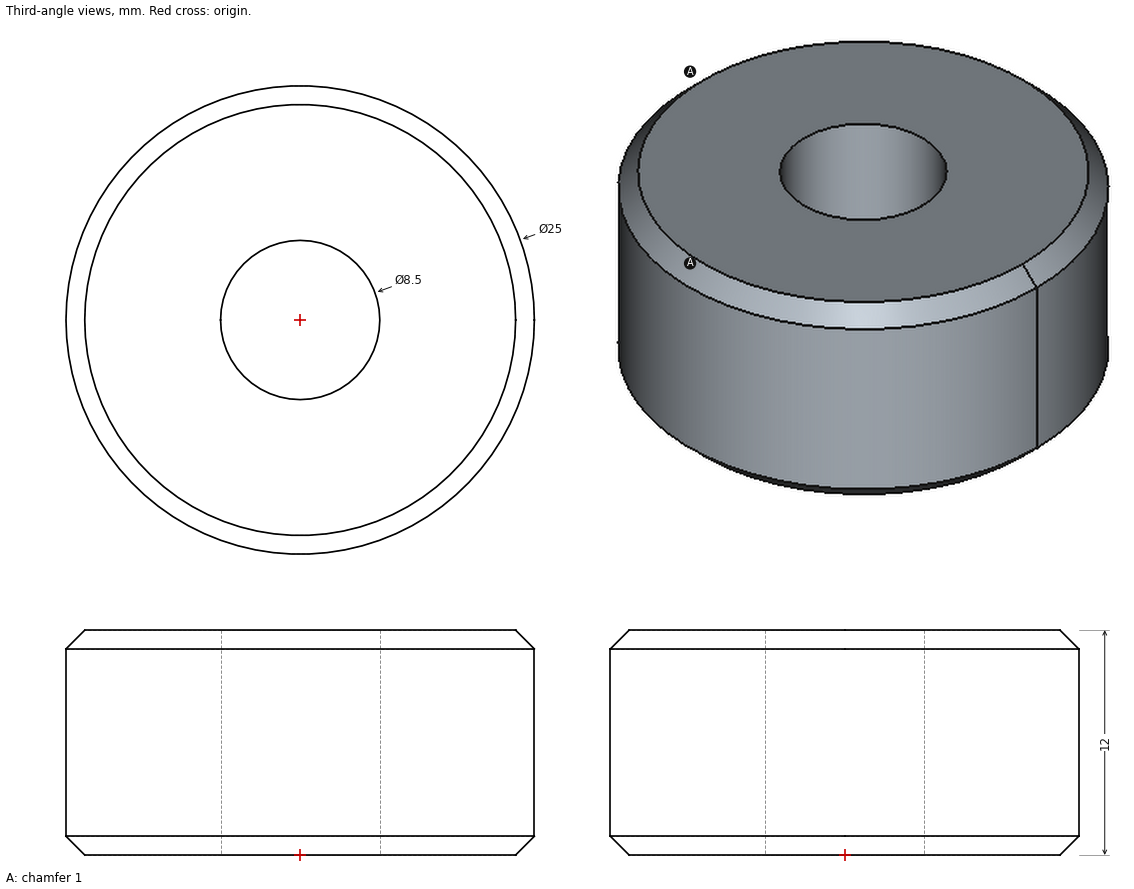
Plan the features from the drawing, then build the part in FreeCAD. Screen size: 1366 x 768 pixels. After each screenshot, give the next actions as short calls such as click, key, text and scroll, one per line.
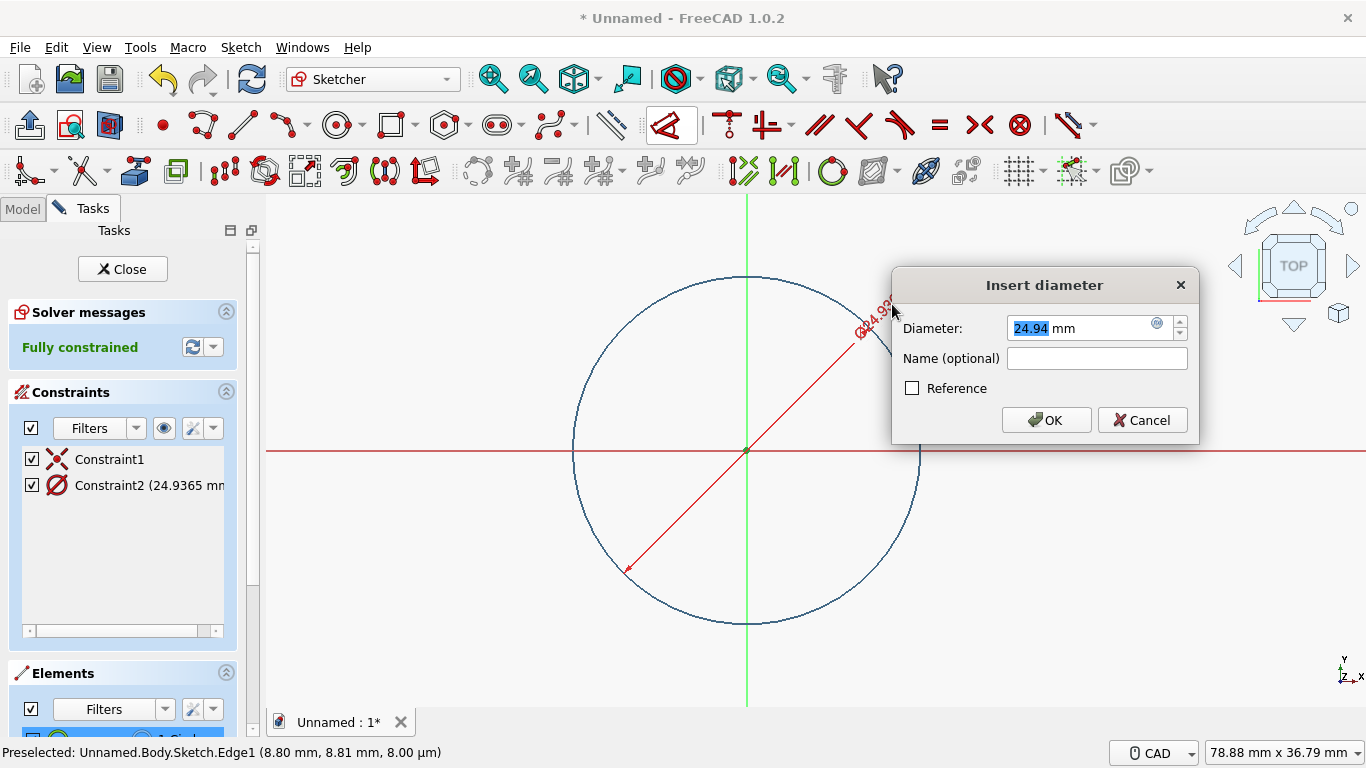
text(25)
key(Return)
key(Escape)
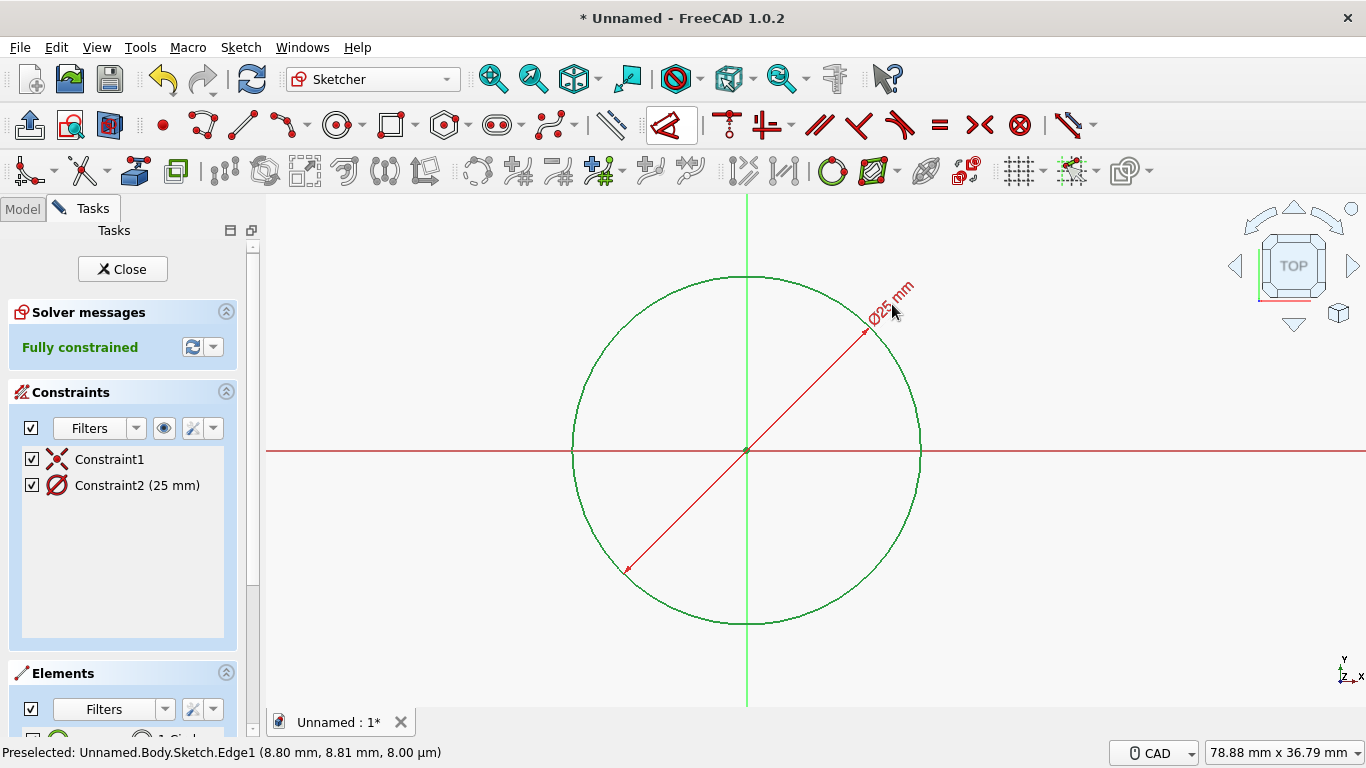
click(123, 269)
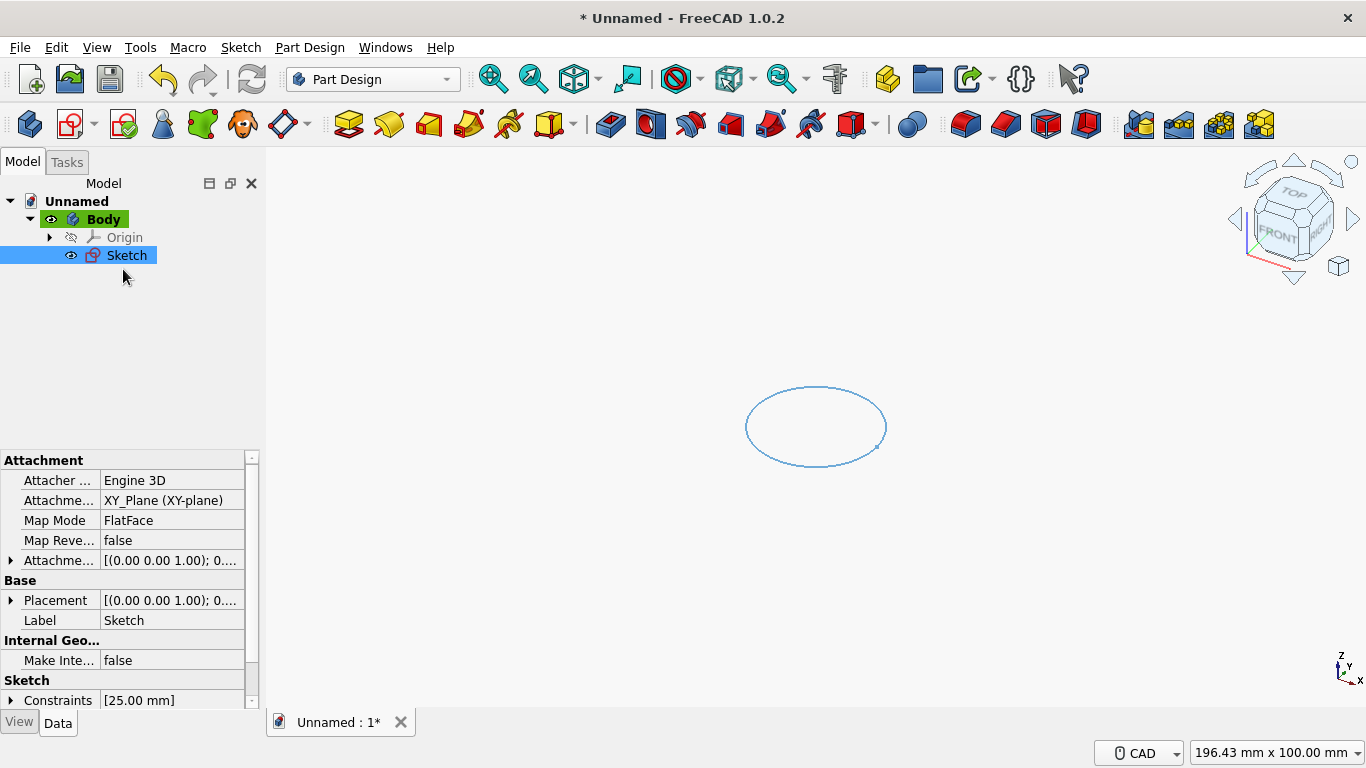
click(350, 124)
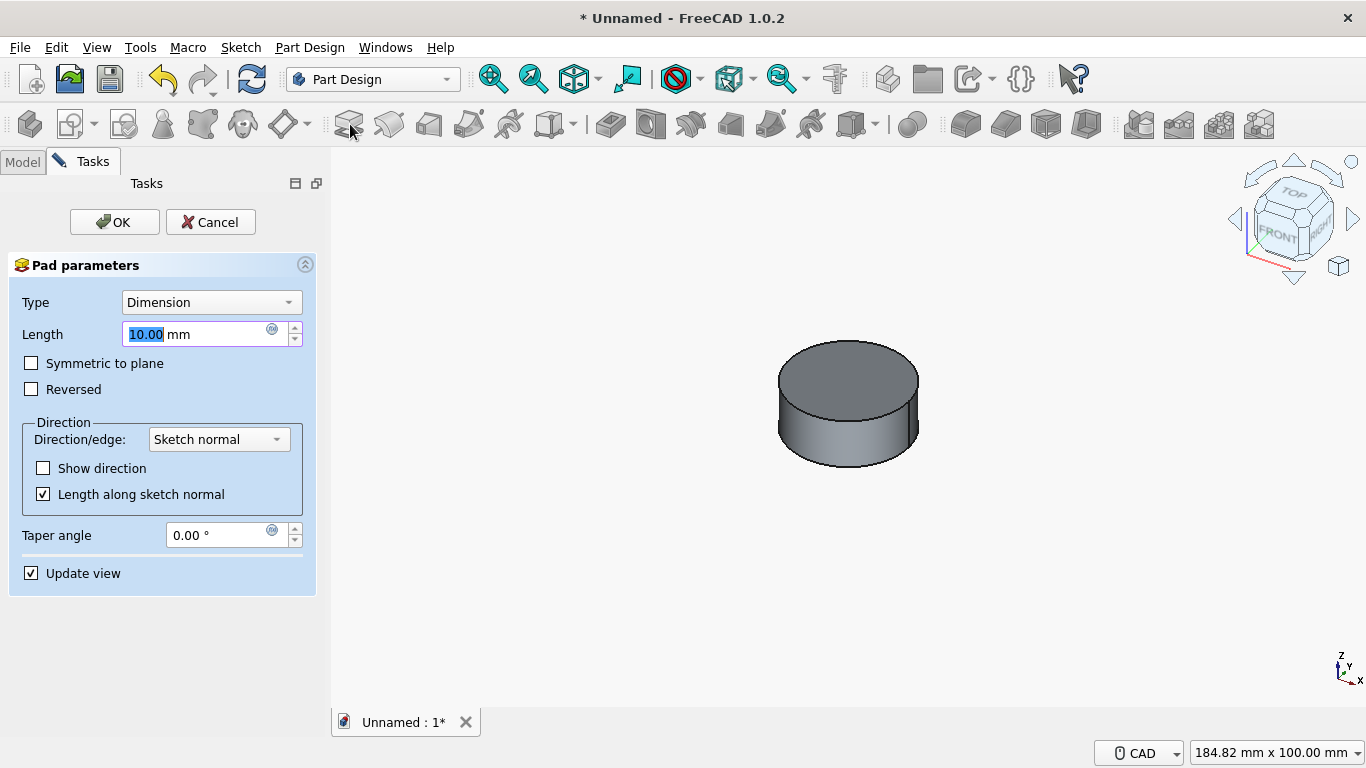
text(12)
key(Tab)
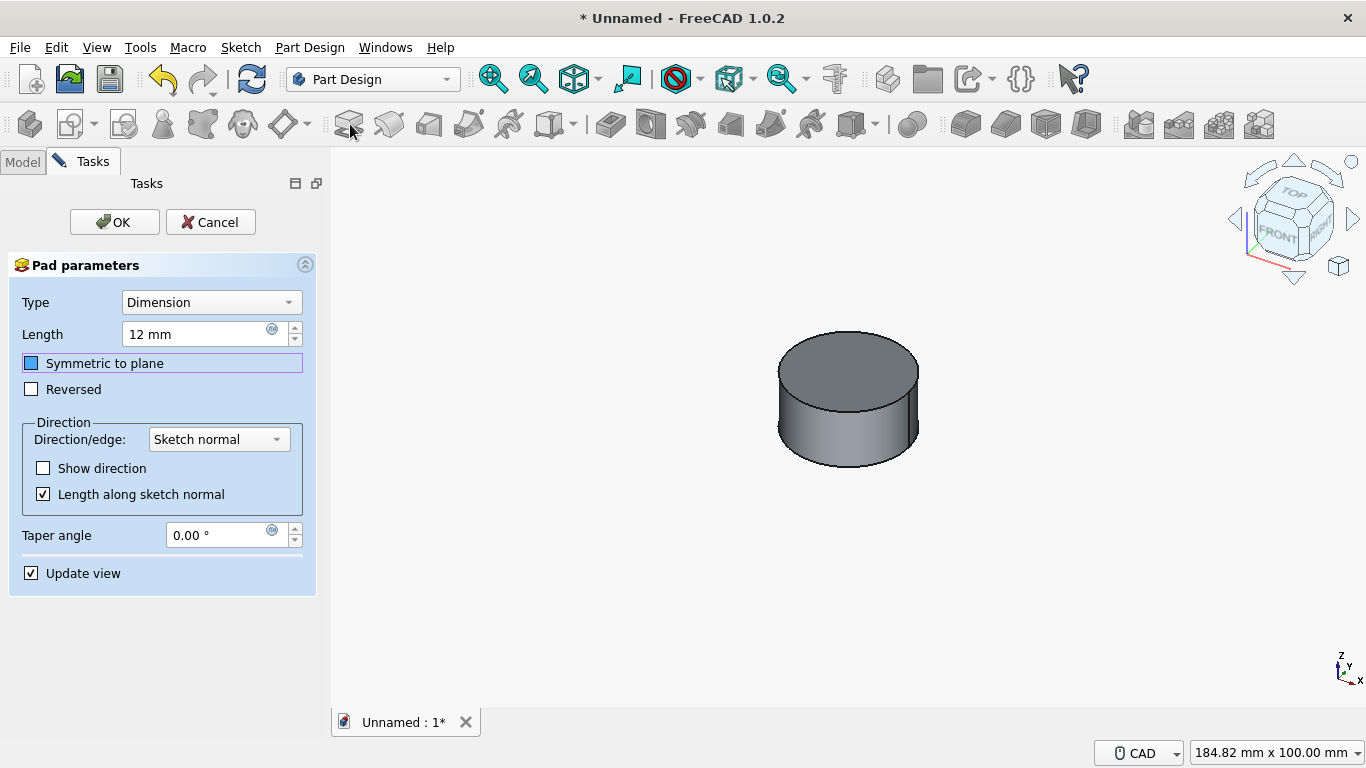
click(115, 222)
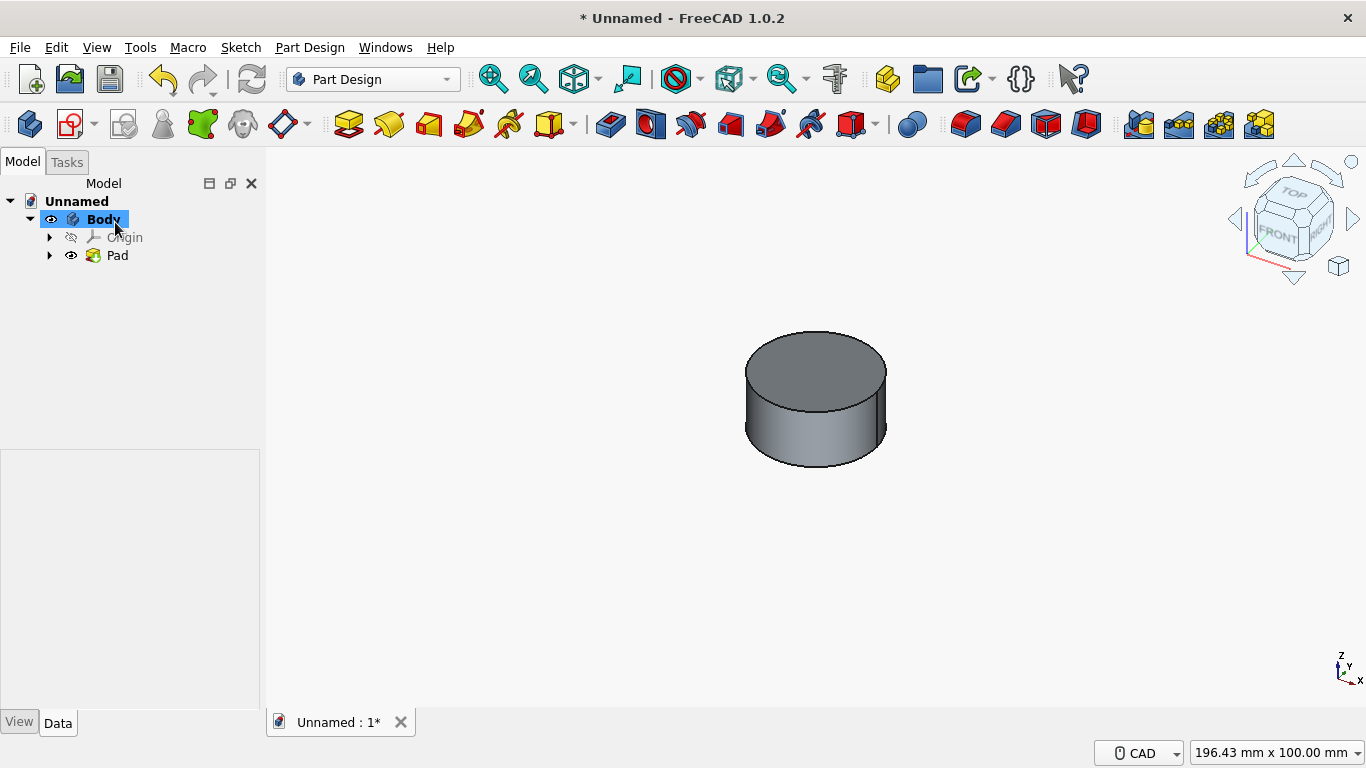
key(v)
key(f)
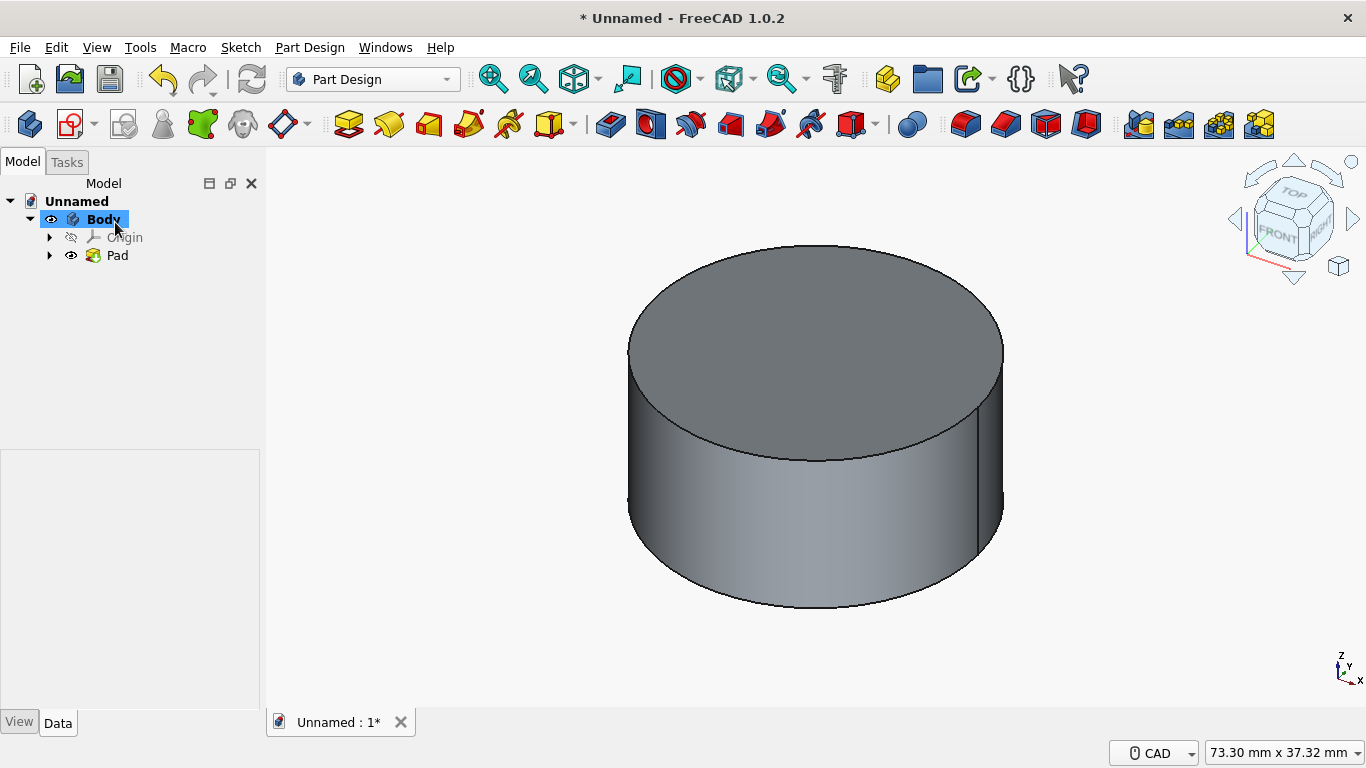
click(816, 352)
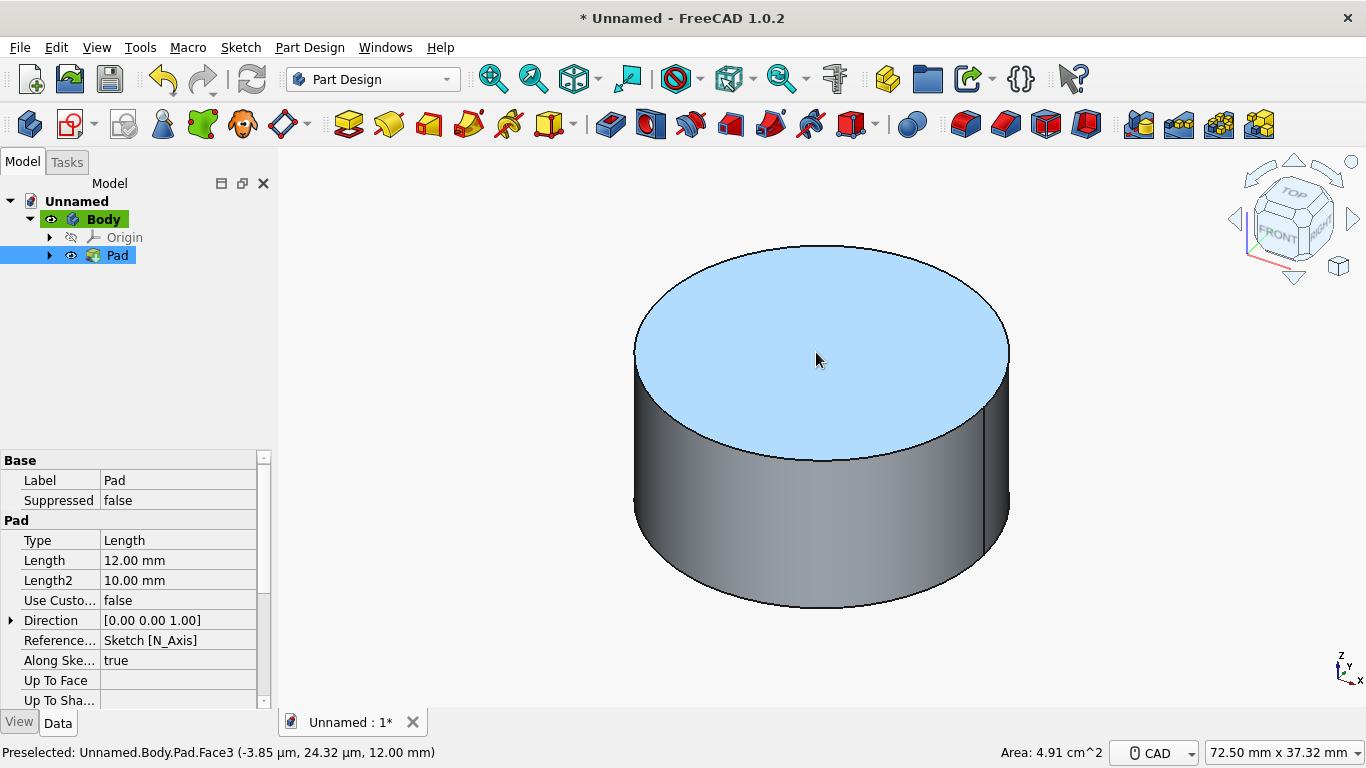
click(70, 124)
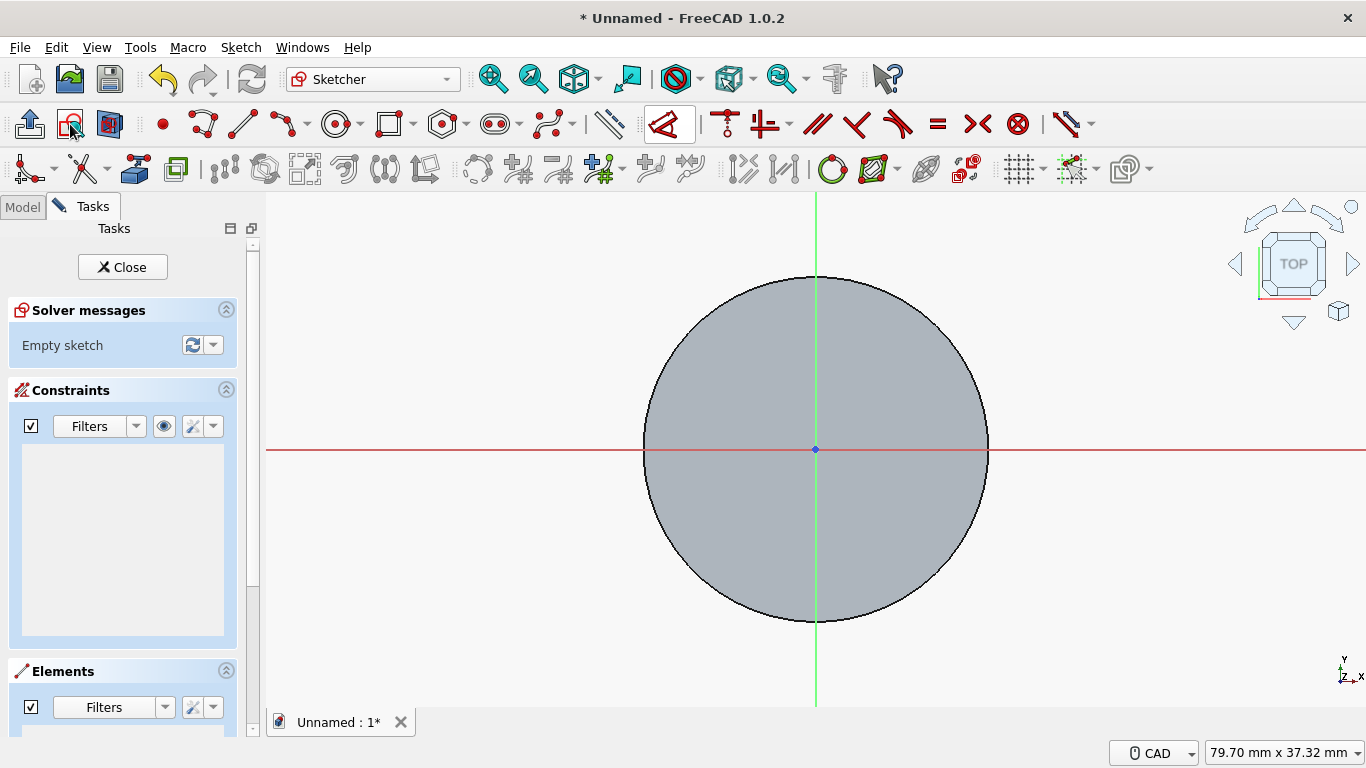
scroll(856, 449, up, 5)